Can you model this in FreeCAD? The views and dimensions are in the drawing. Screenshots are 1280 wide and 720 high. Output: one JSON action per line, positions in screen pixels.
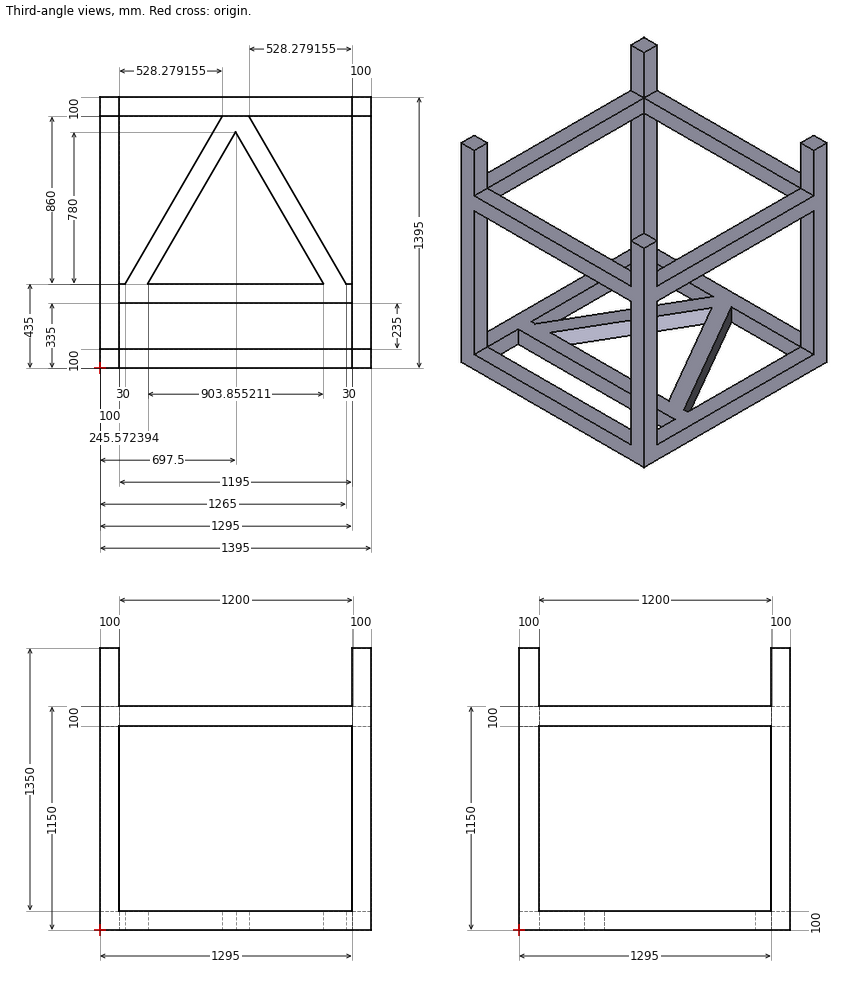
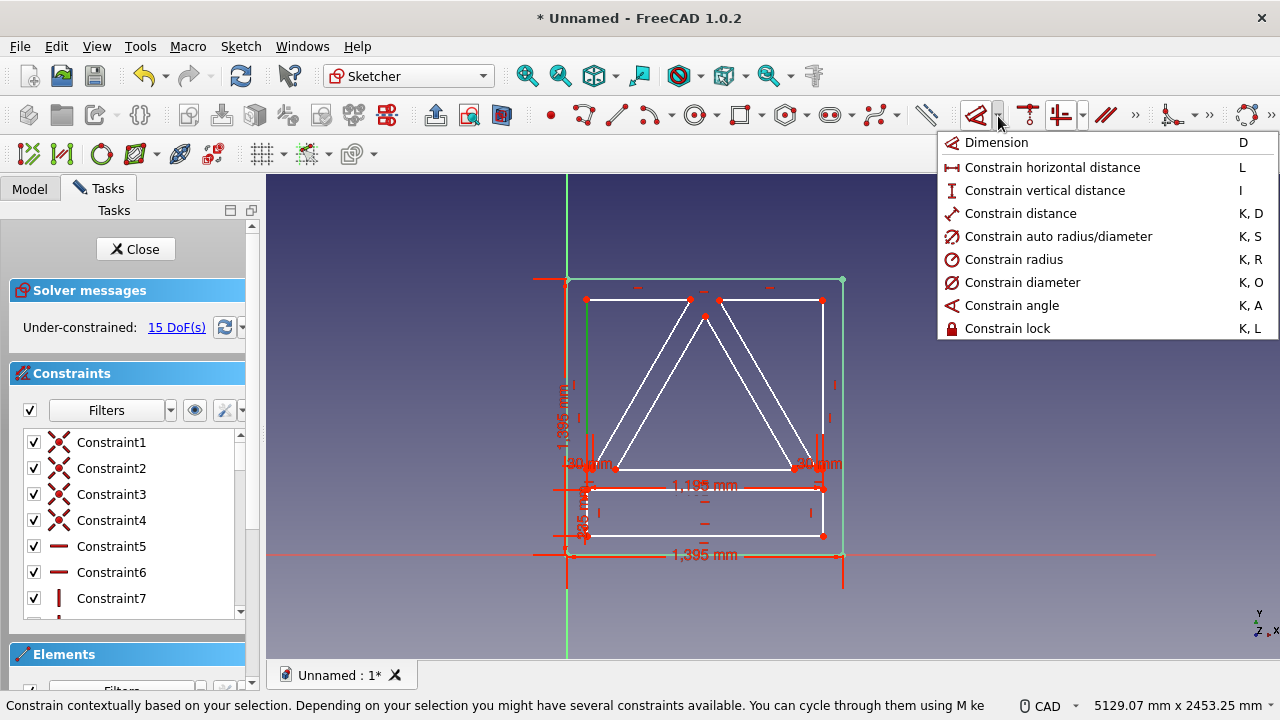
{"action": "left_click", "coordinate": [1108, 190]}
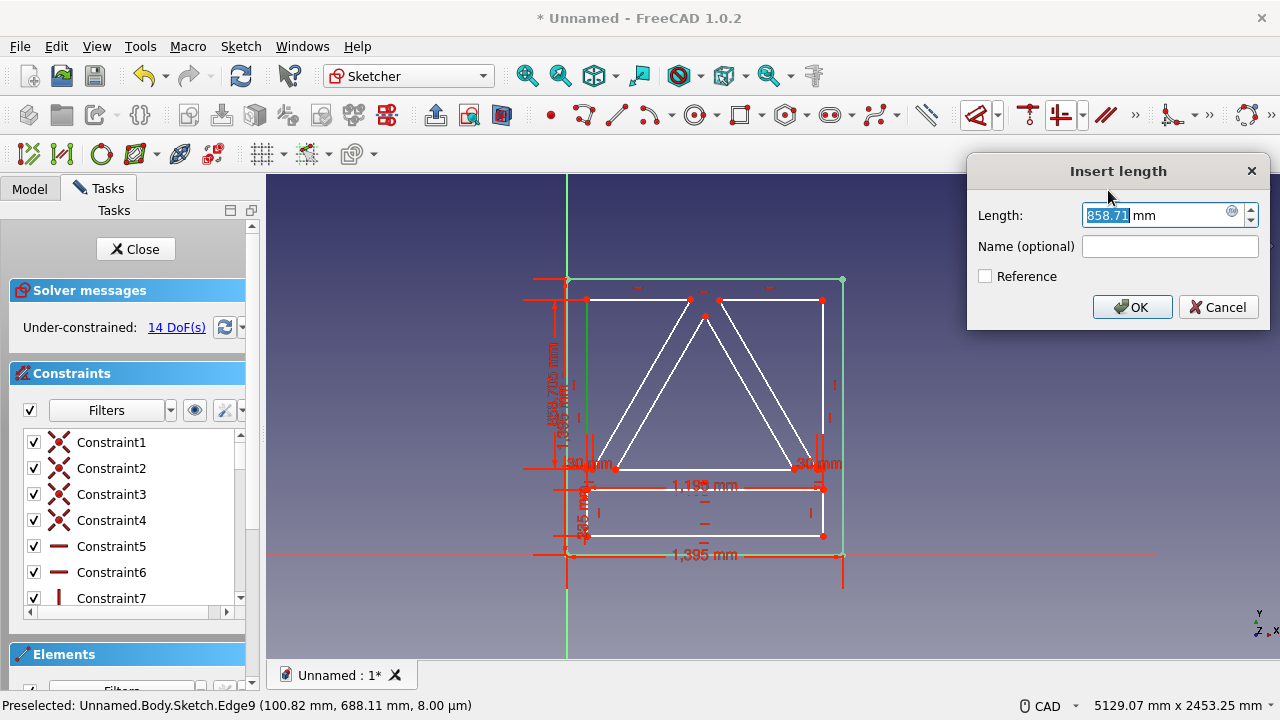
{"action": "type", "text": "860"}
{"action": "key", "text": "Return"}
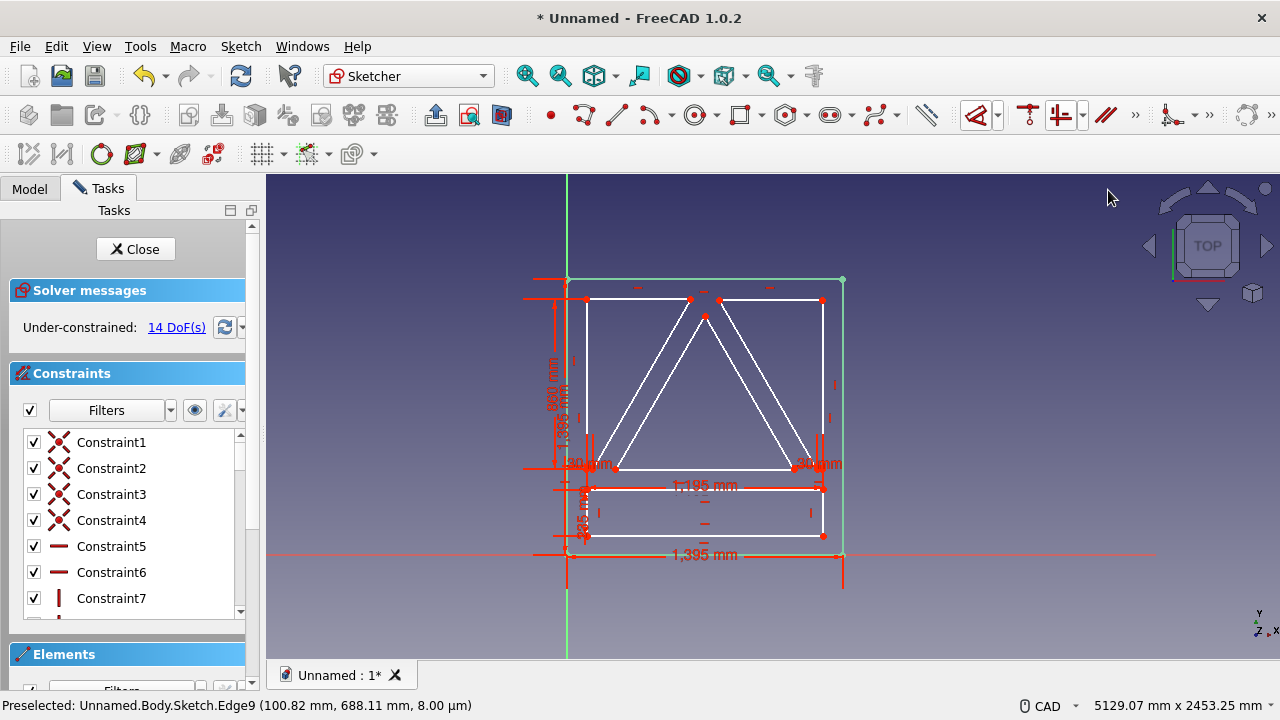
{"action": "left_click", "coordinate": [823, 351]}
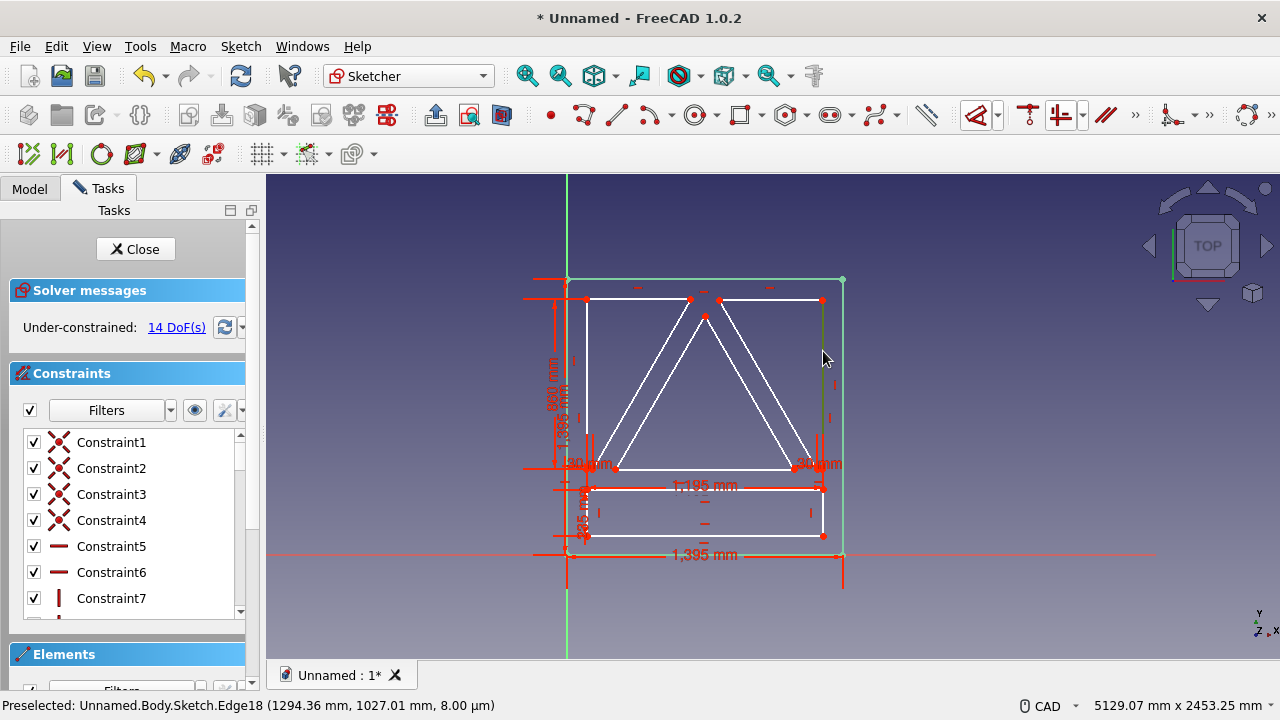
{"action": "key", "text": "i"}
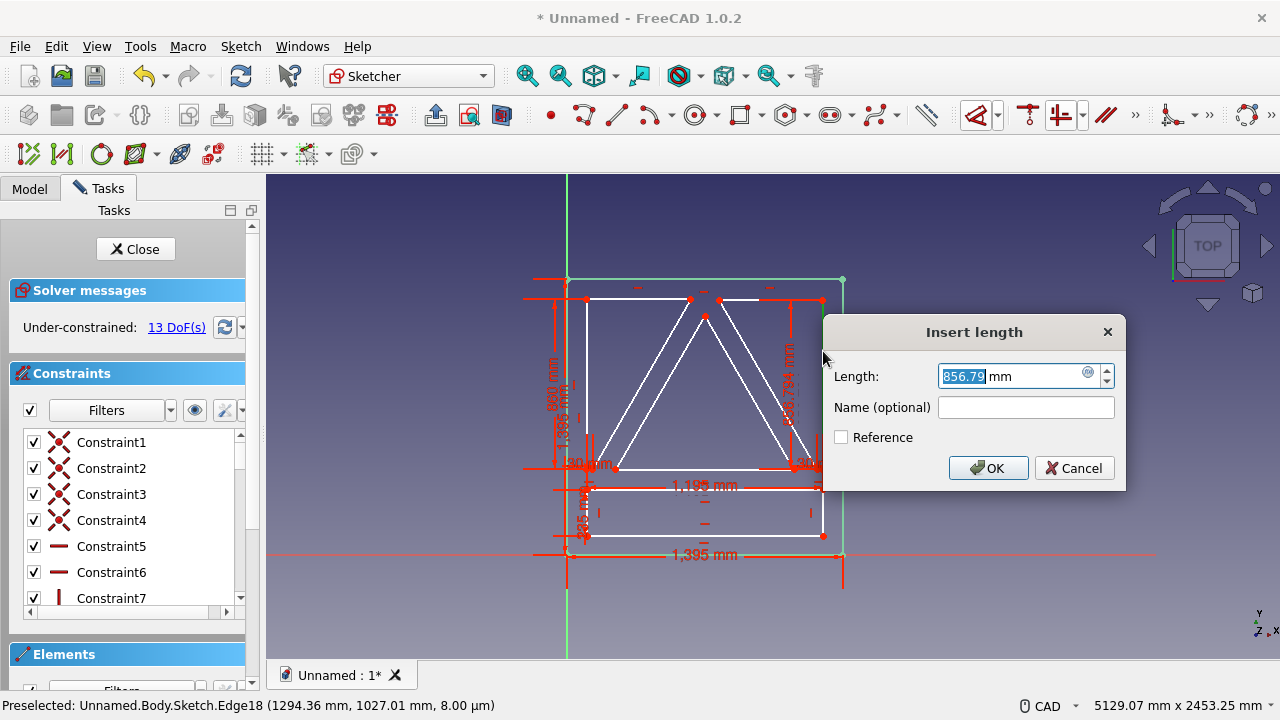
{"action": "type", "text": "860"}
{"action": "key", "text": "Return"}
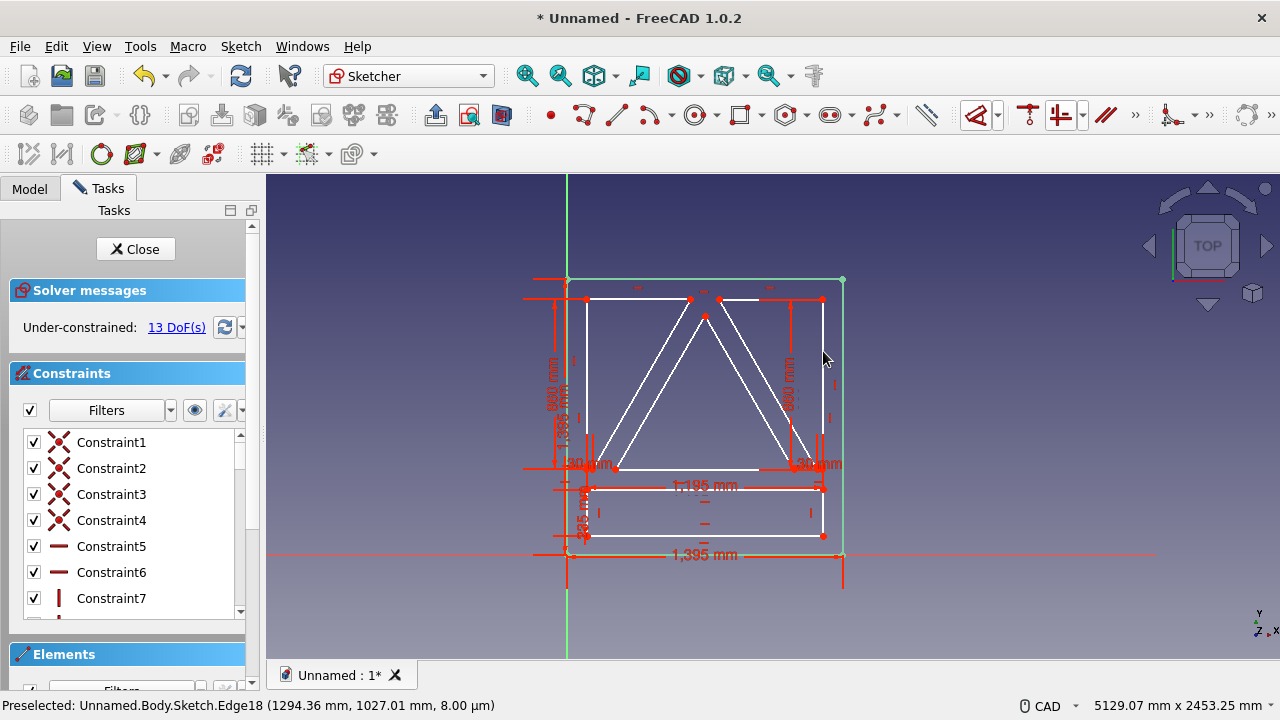
{"action": "scroll", "coordinate": [587, 490], "scroll_direction": "up", "scroll_amount": 4}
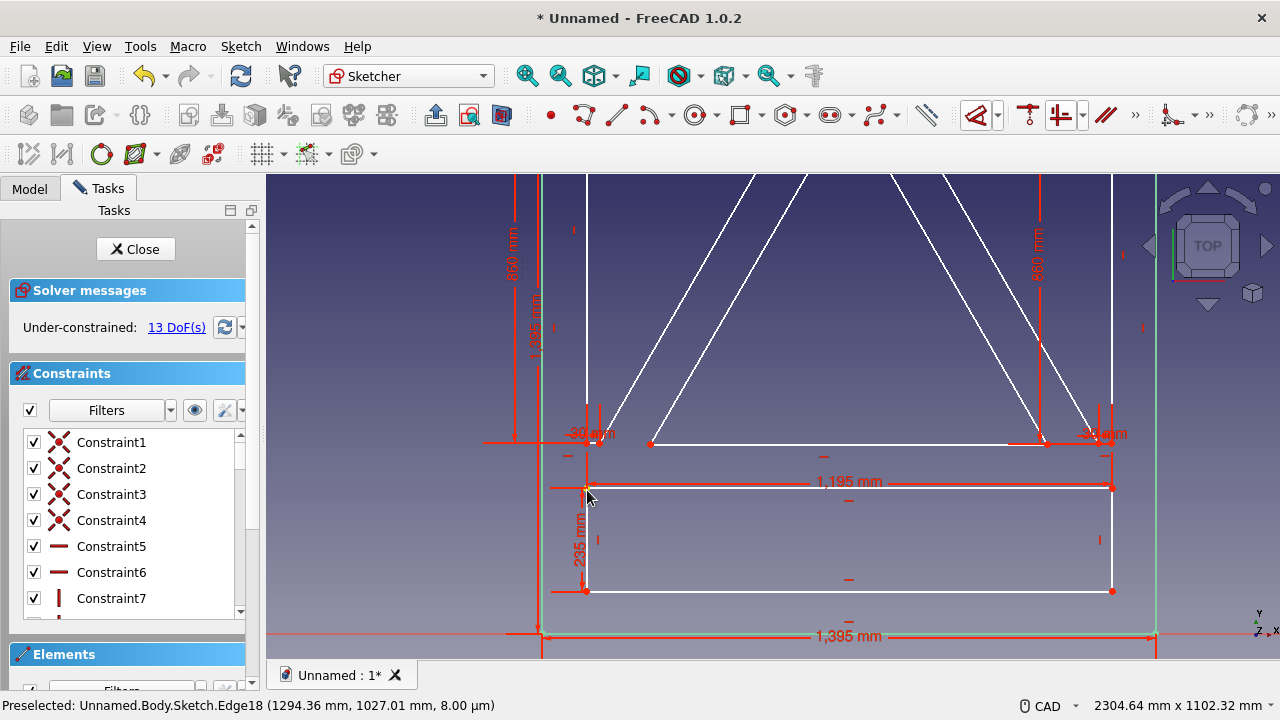
{"action": "left_click", "coordinate": [587, 488]}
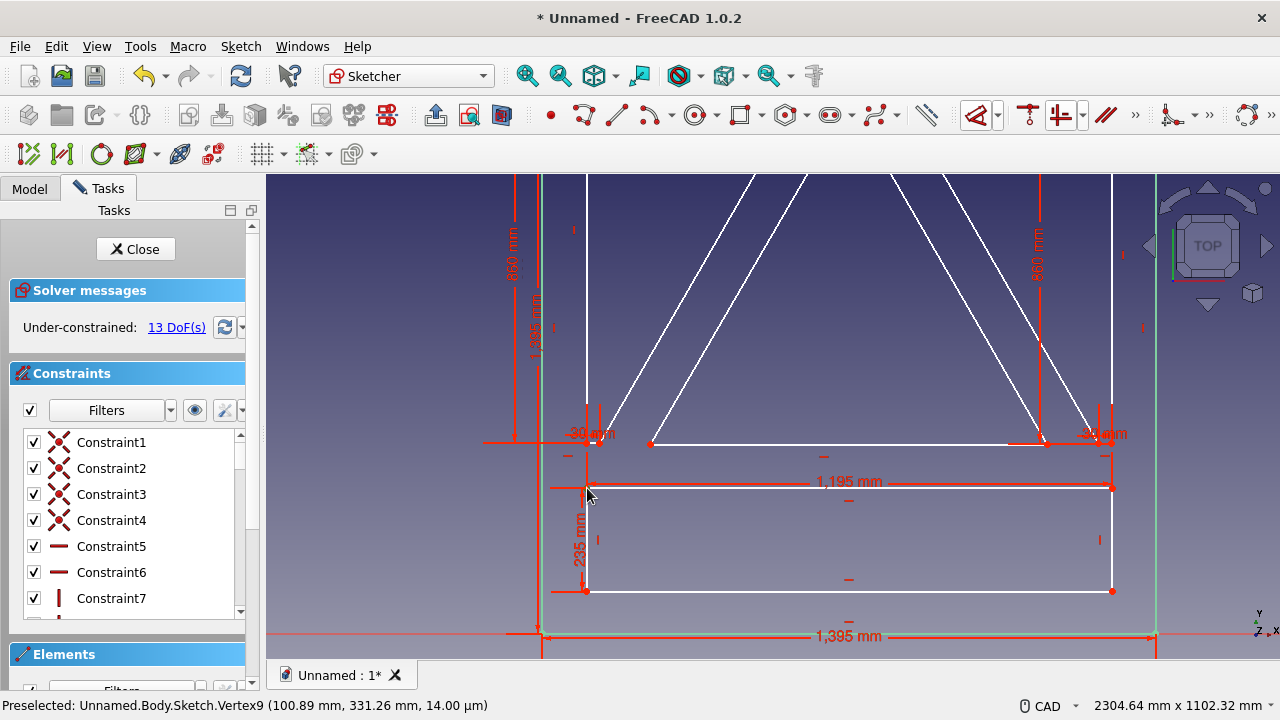
{"action": "key", "text": "l"}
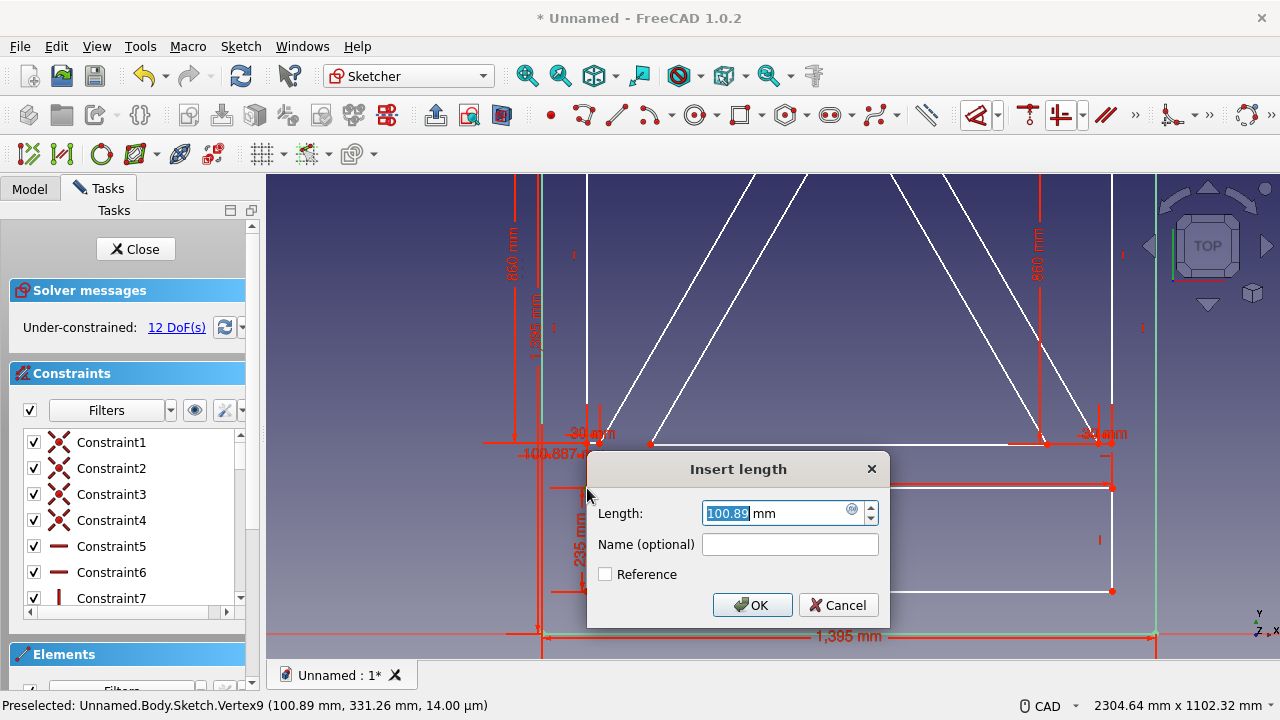
{"action": "type", "text": "100"}
{"action": "key", "text": "Return"}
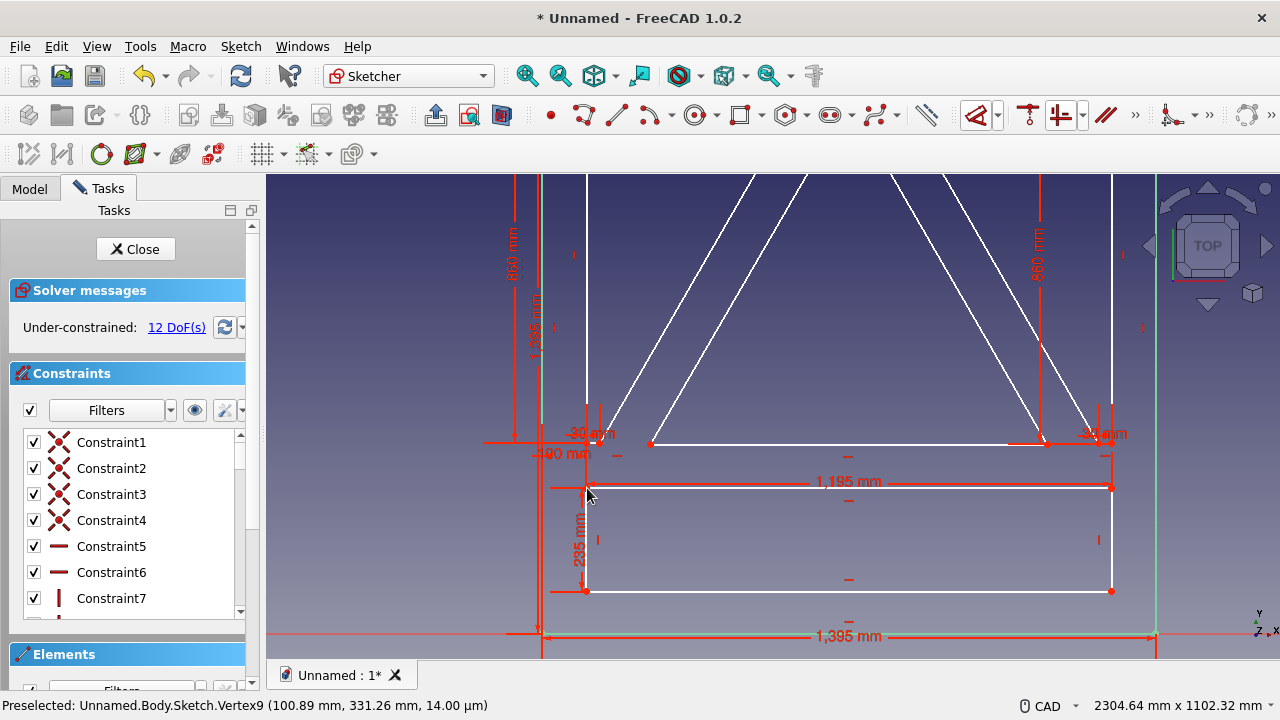
{"action": "left_click", "coordinate": [586, 488]}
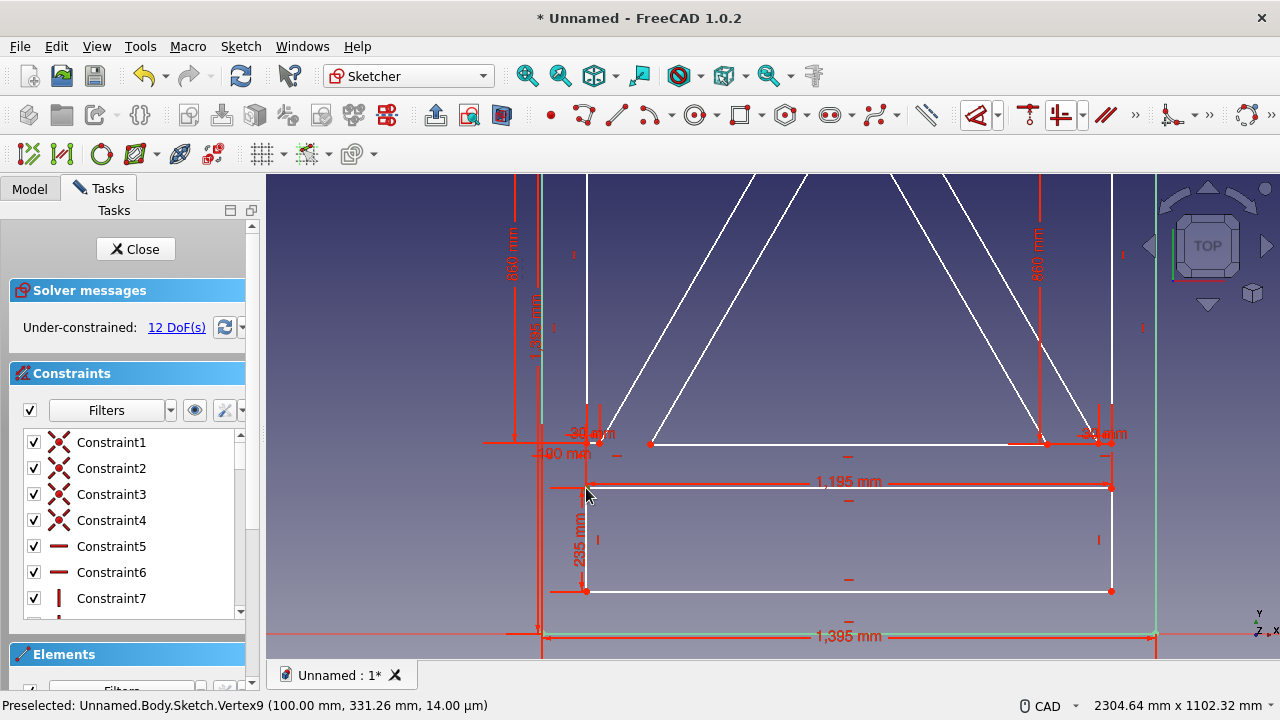
{"action": "key", "text": "i"}